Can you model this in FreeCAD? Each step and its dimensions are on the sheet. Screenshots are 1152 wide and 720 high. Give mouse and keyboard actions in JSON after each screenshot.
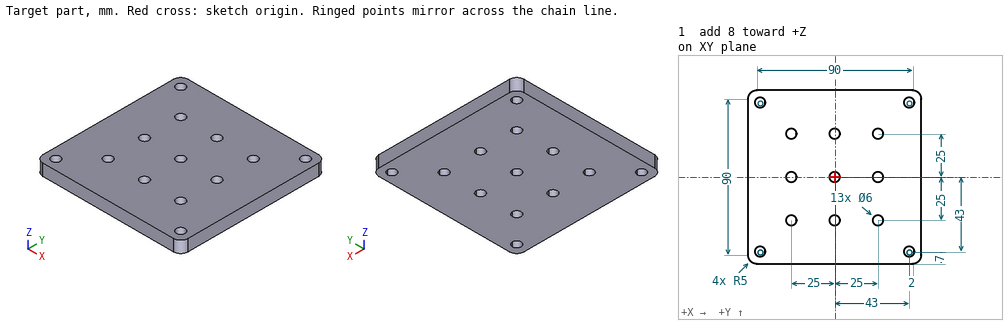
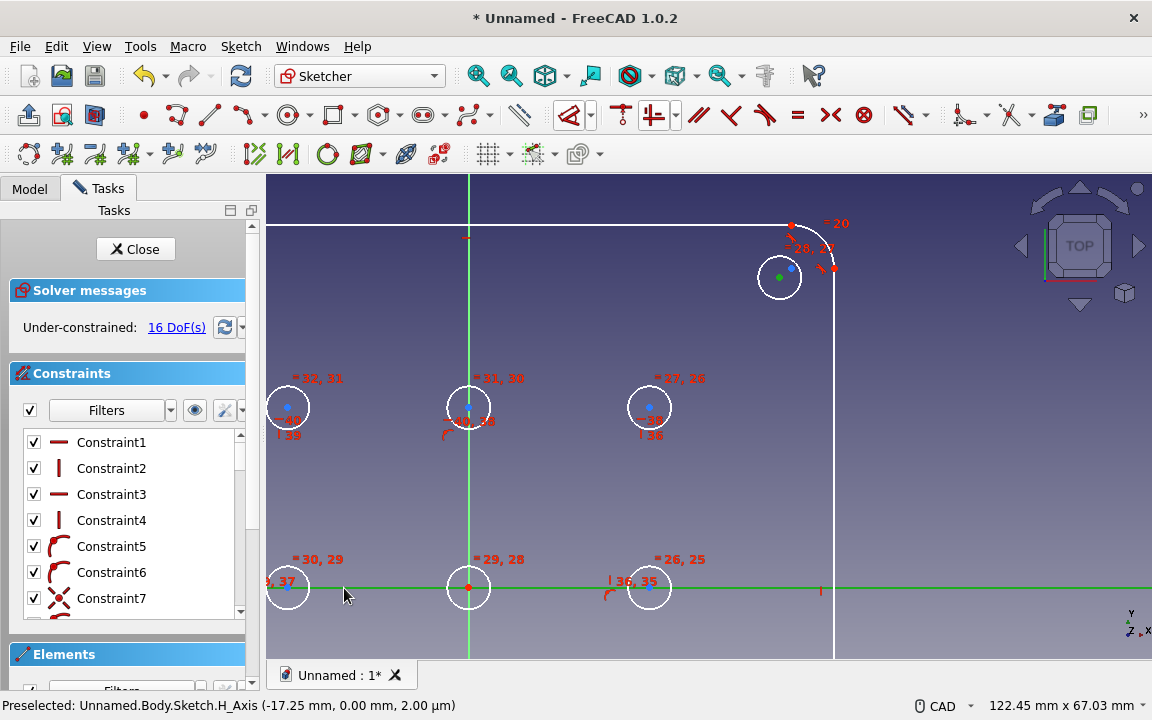
{"action": "left_click", "coordinate": [831, 116]}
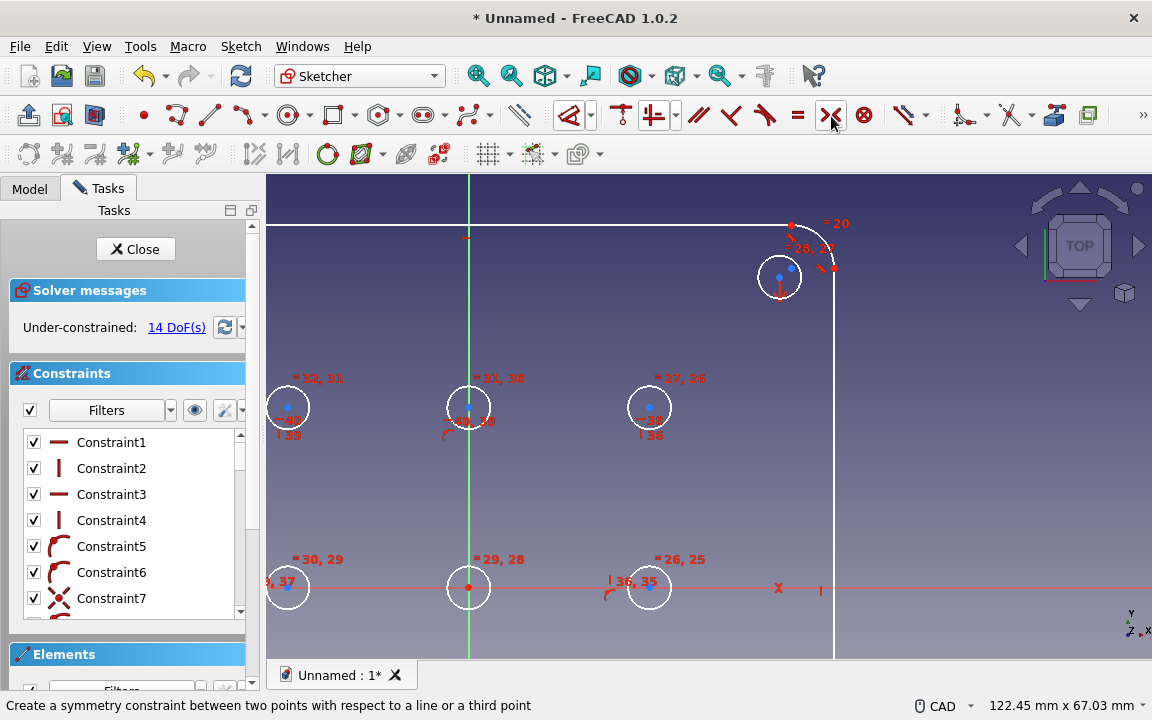
{"action": "scroll", "coordinate": [781, 277], "scroll_direction": "down", "scroll_amount": 4}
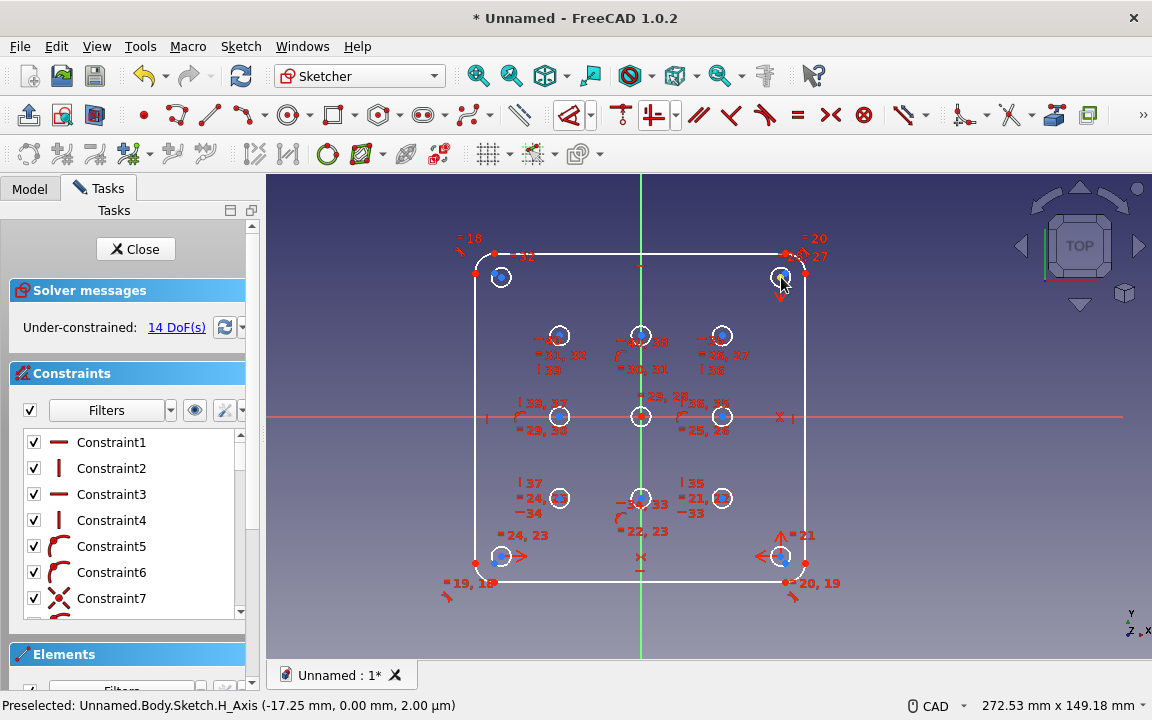
{"action": "scroll", "coordinate": [501, 556], "scroll_direction": "up", "scroll_amount": 2}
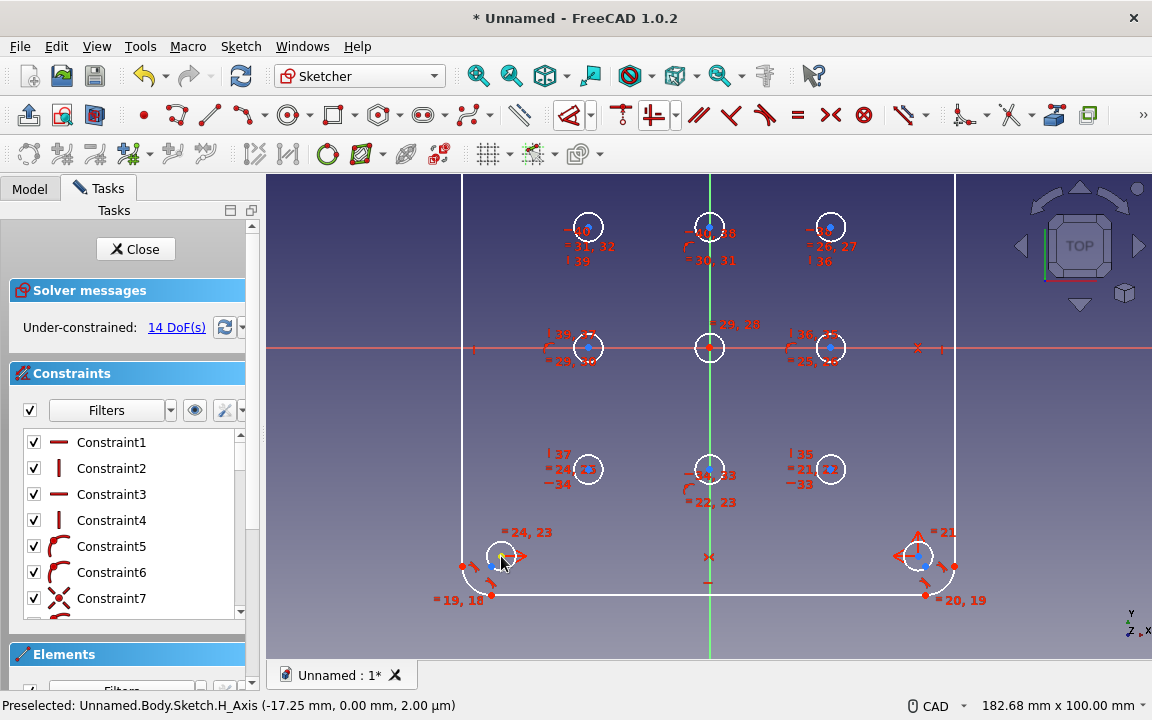
{"action": "left_click", "coordinate": [501, 556]}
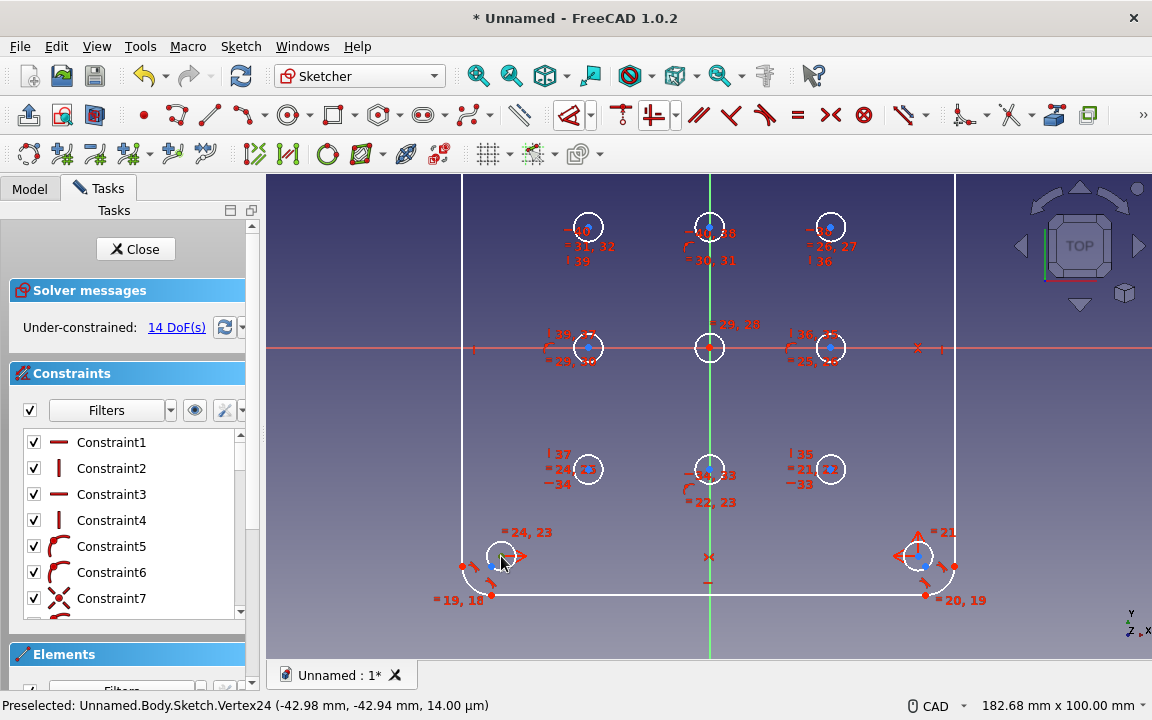
{"action": "scroll", "coordinate": [500, 556], "scroll_direction": "down", "scroll_amount": 2}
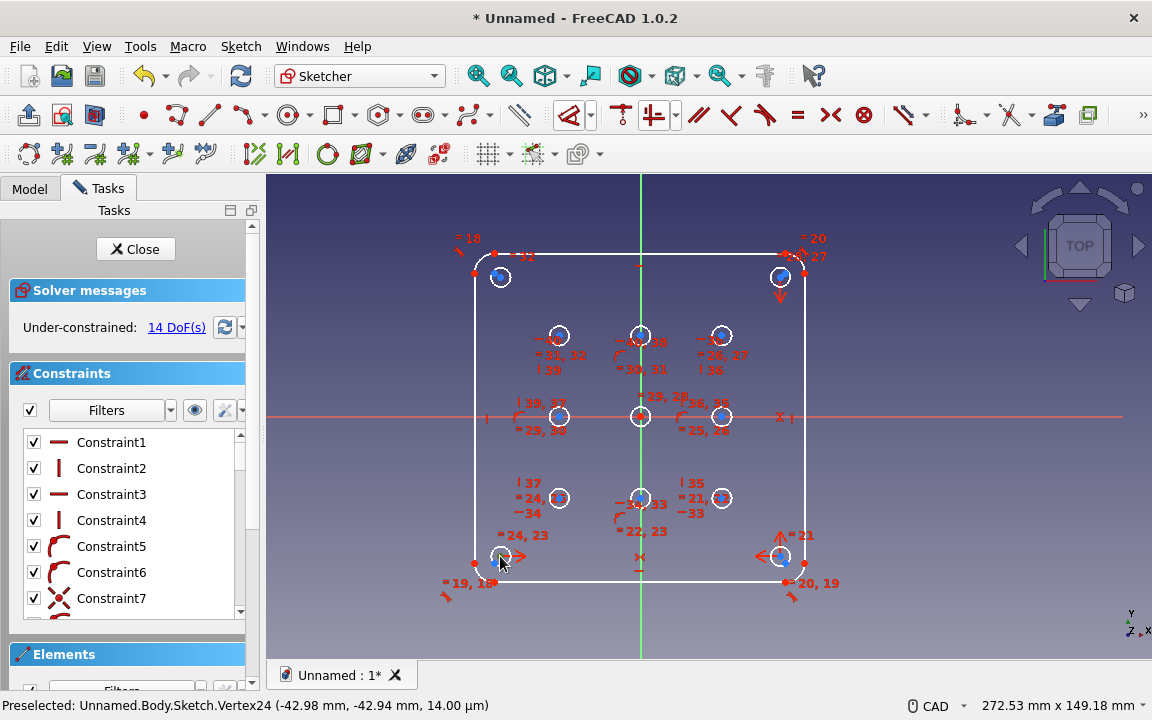
{"action": "scroll", "coordinate": [501, 277], "scroll_direction": "up", "scroll_amount": 3}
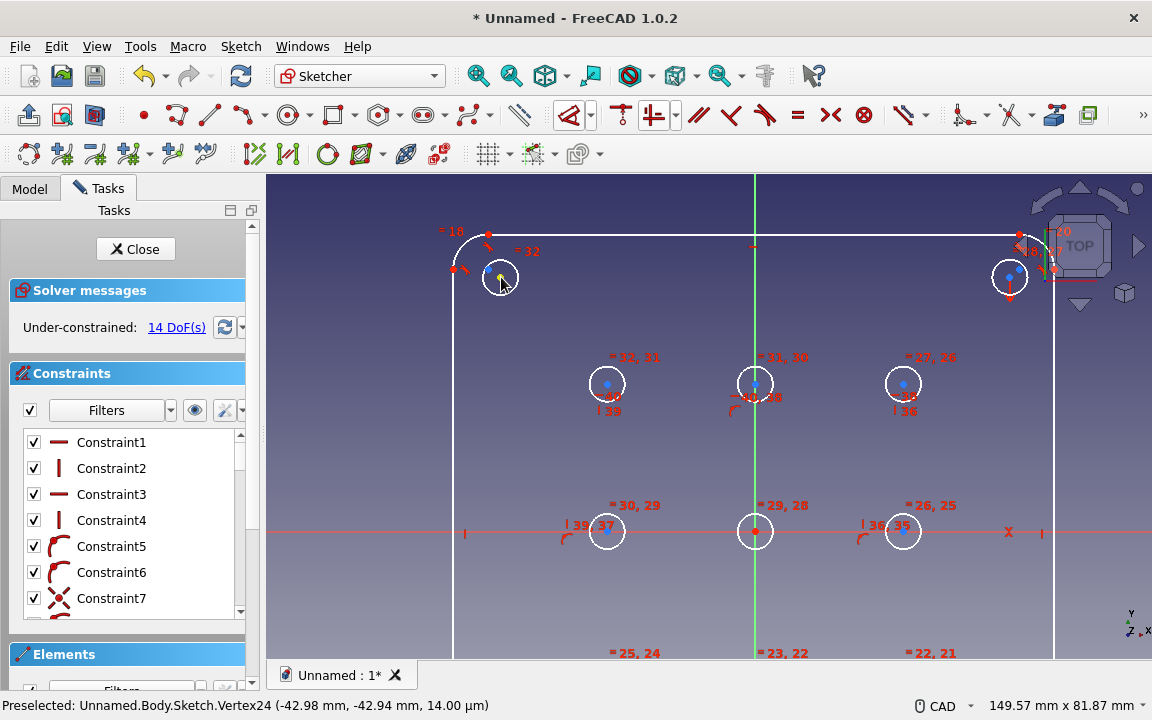
{"action": "left_click", "coordinate": [501, 278]}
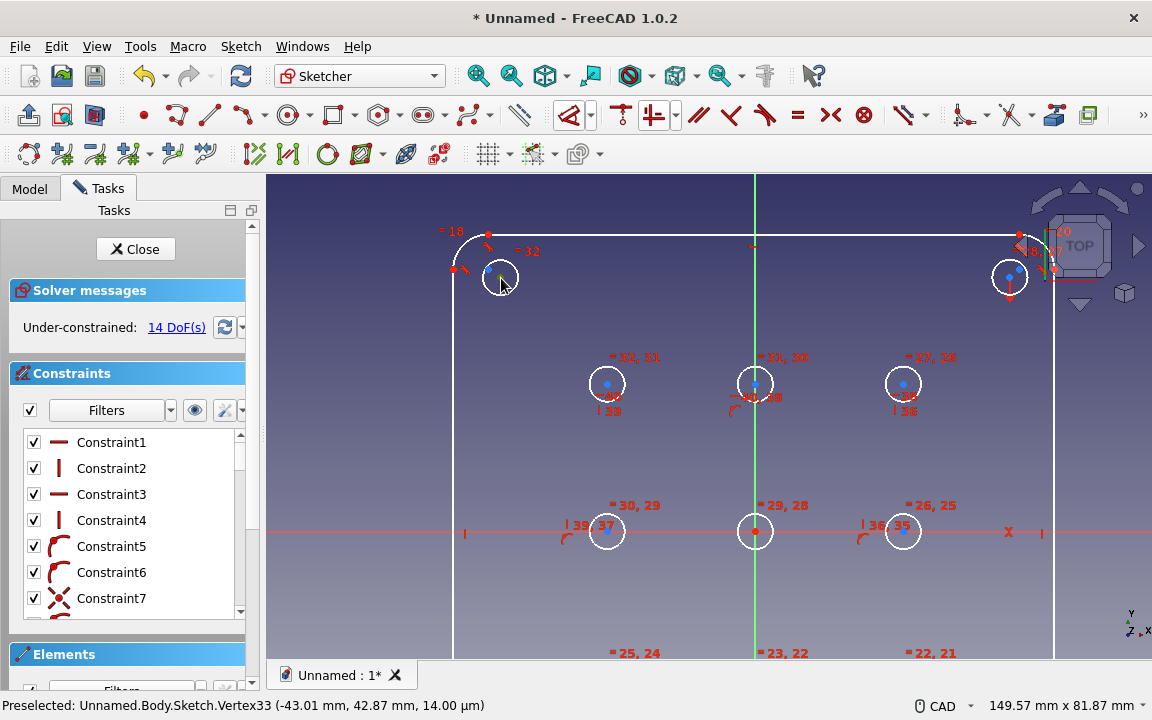
{"action": "left_click", "coordinate": [344, 532]}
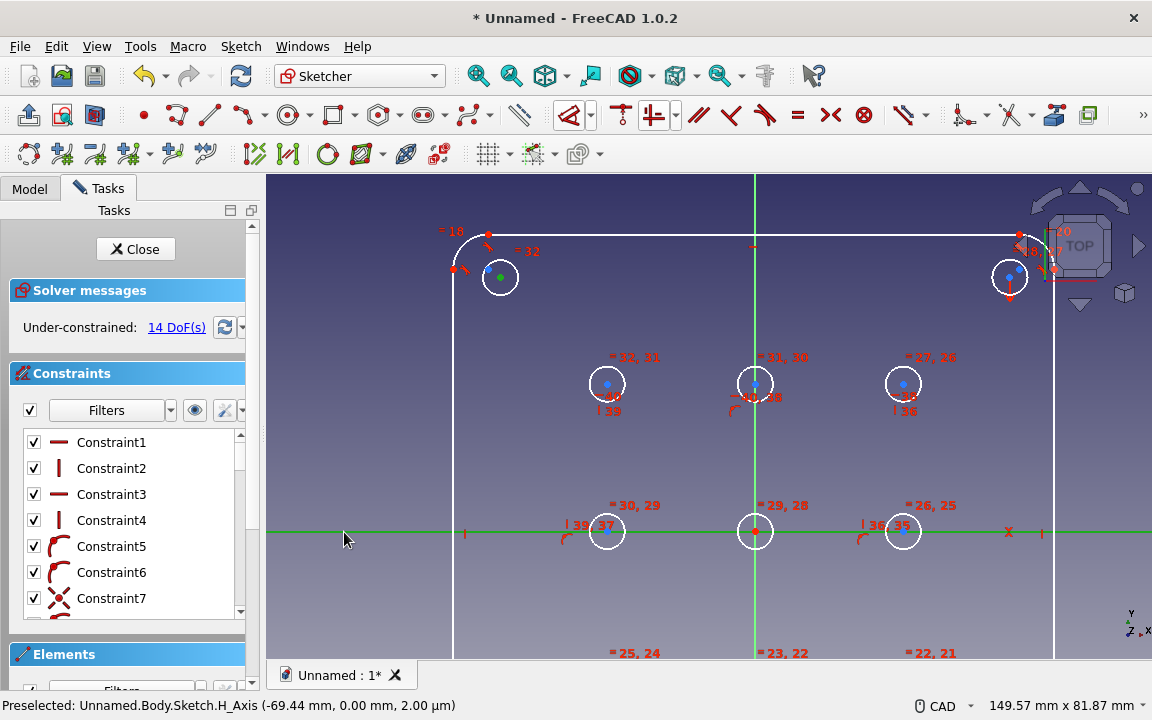
{"action": "left_click", "coordinate": [831, 116]}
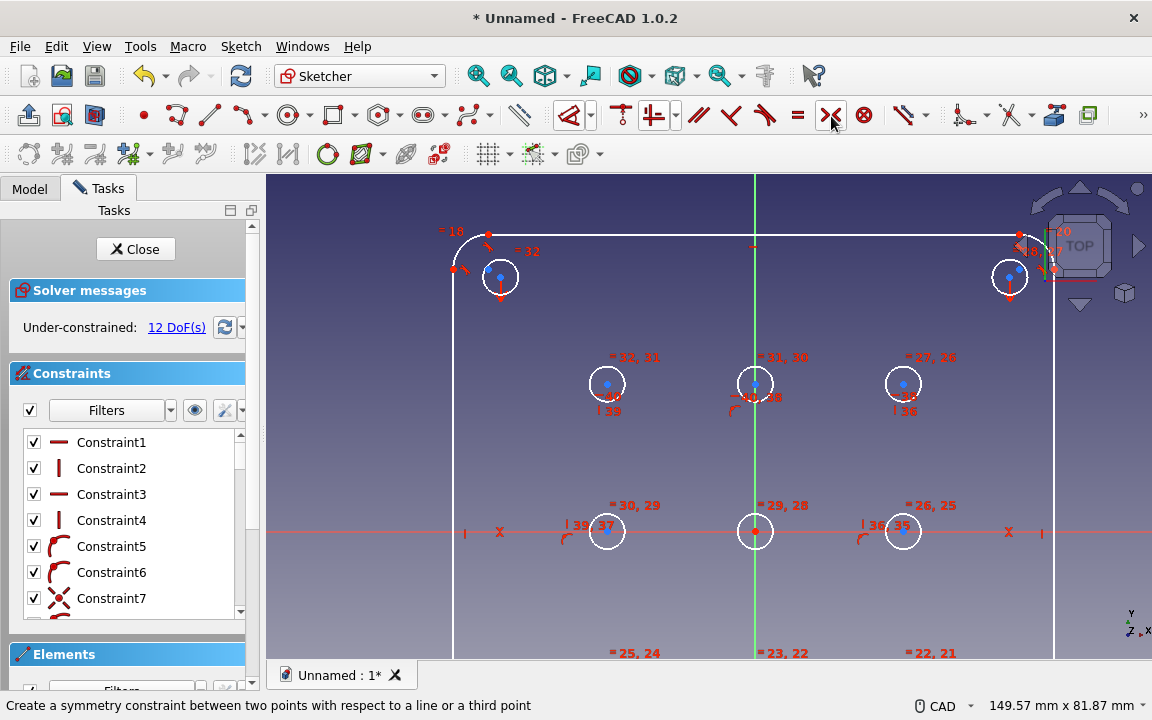
{"action": "scroll", "coordinate": [472, 238], "scroll_direction": "up", "scroll_amount": 2}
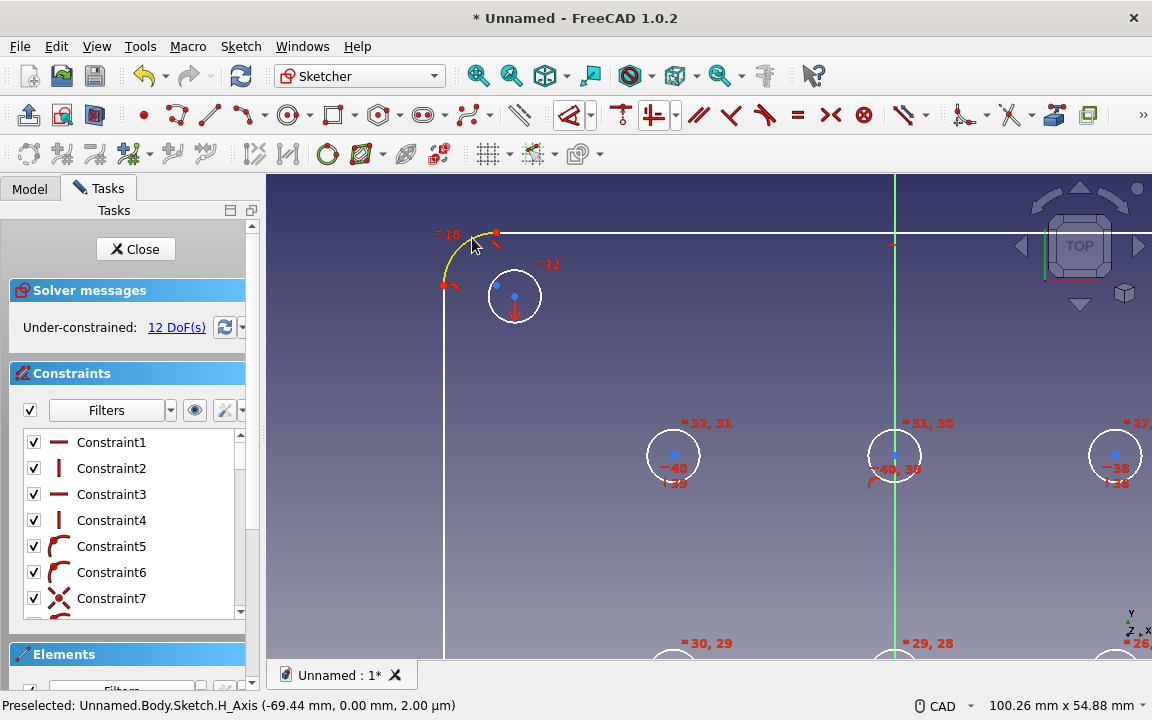
{"action": "left_click", "coordinate": [473, 238]}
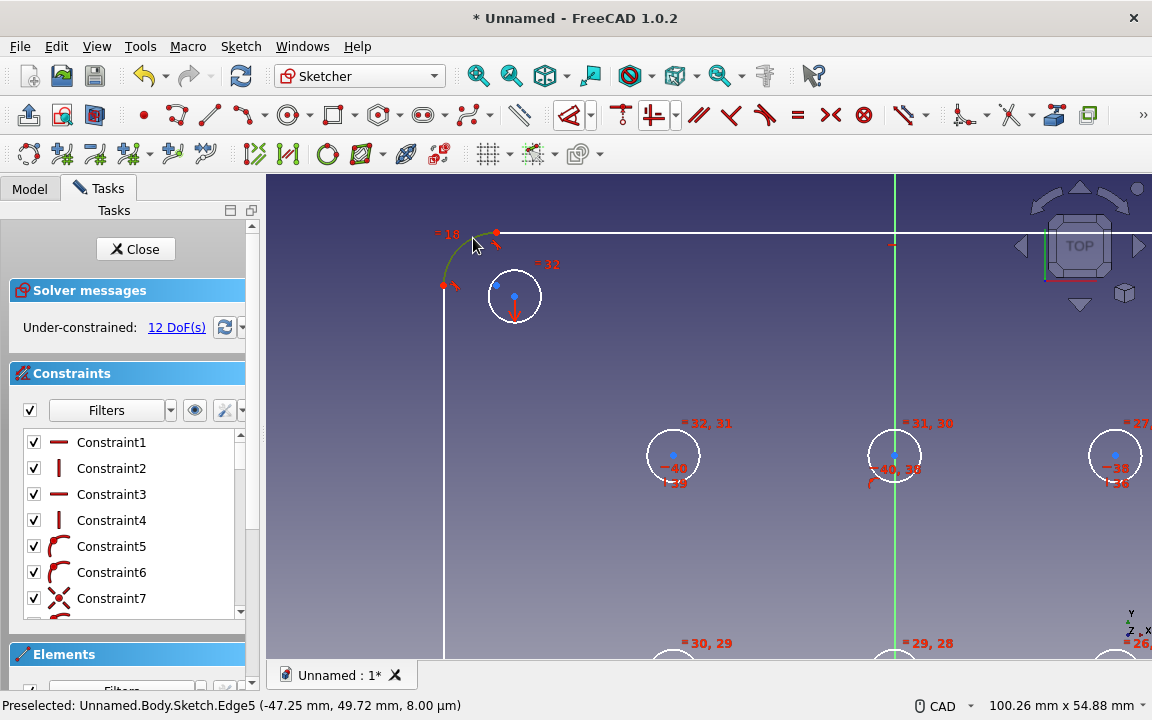
{"action": "key", "text": "k r"}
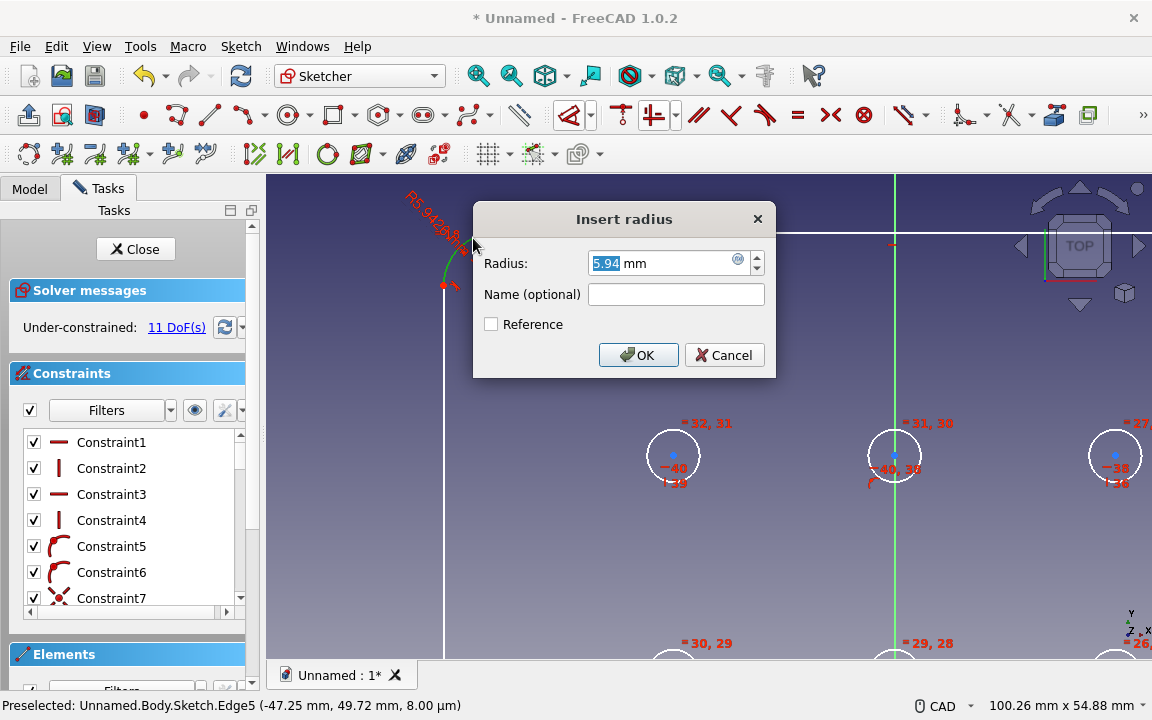
{"action": "type", "text": "5"}
{"action": "key", "text": "Return"}